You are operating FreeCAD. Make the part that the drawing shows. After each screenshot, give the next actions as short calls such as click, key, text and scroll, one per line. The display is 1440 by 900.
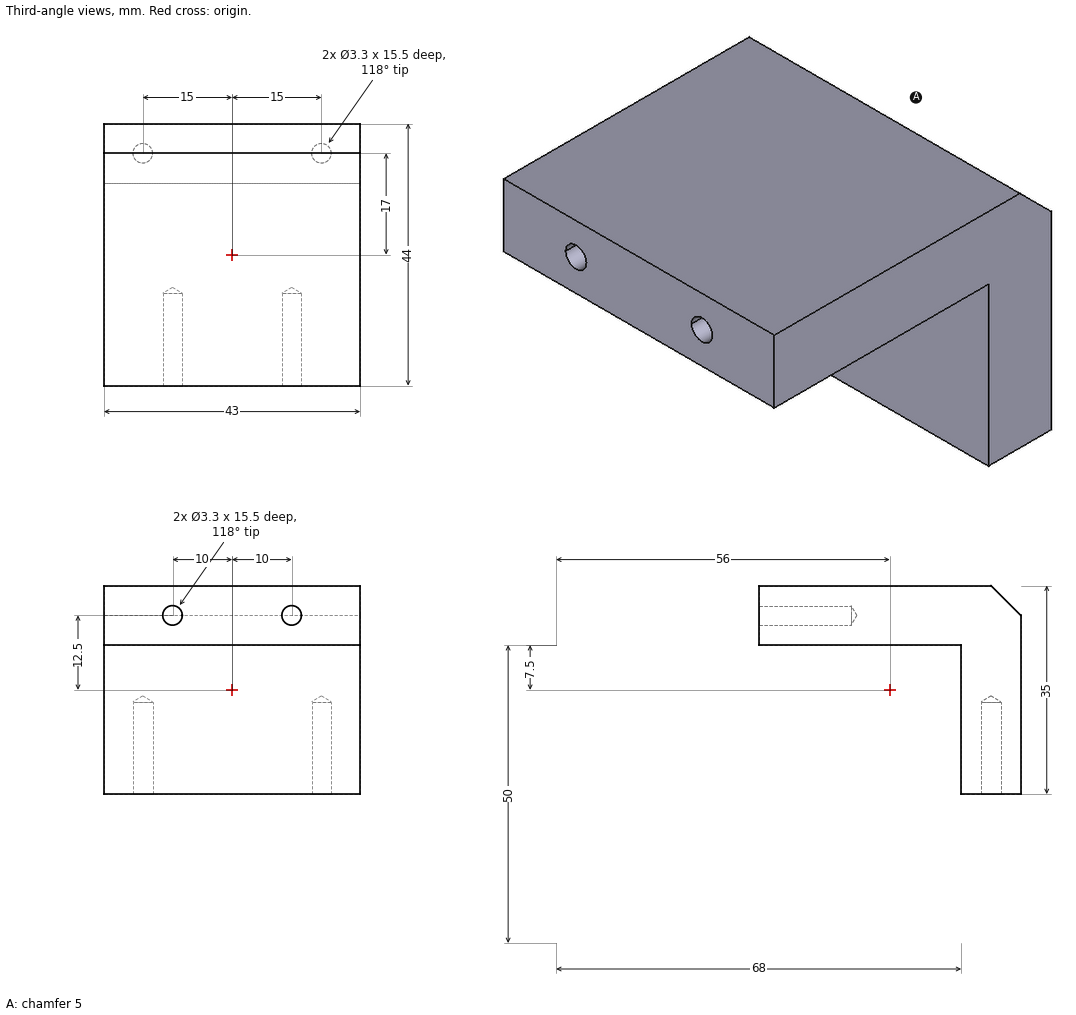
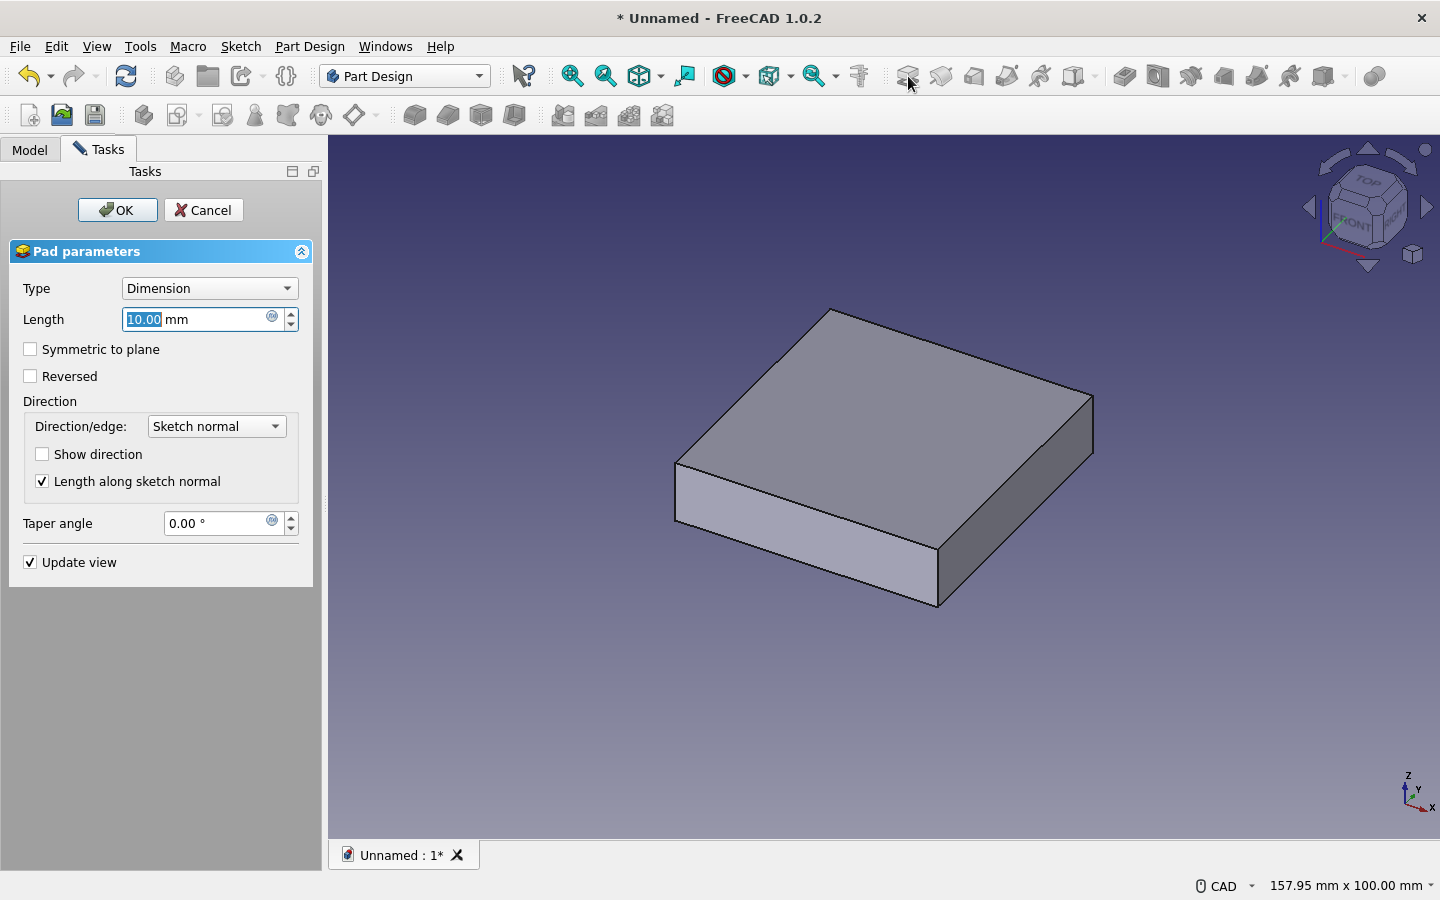
text(35)
key(Tab)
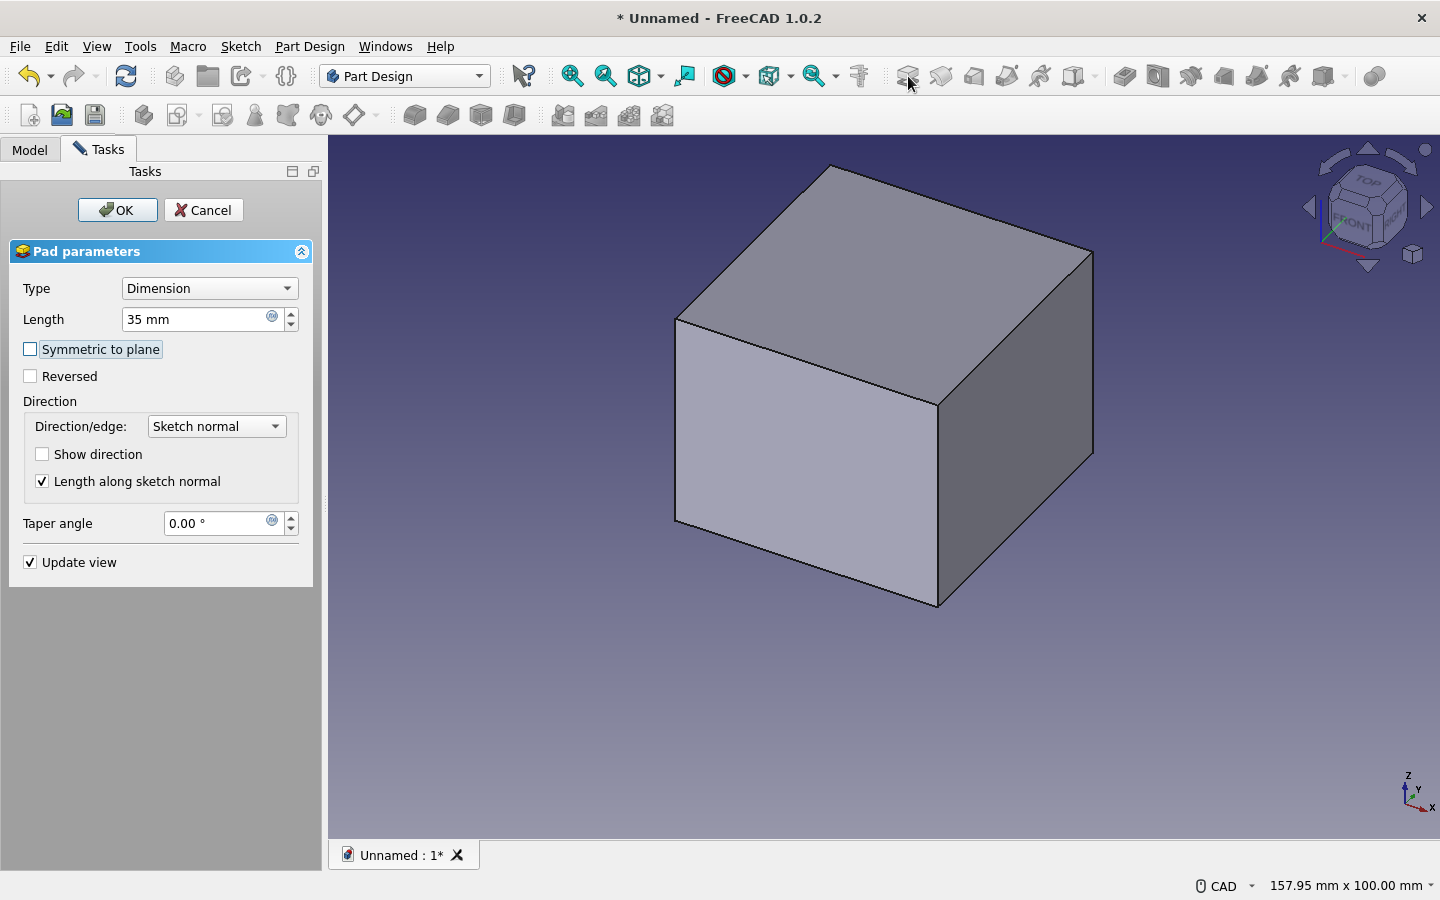
click(31, 349)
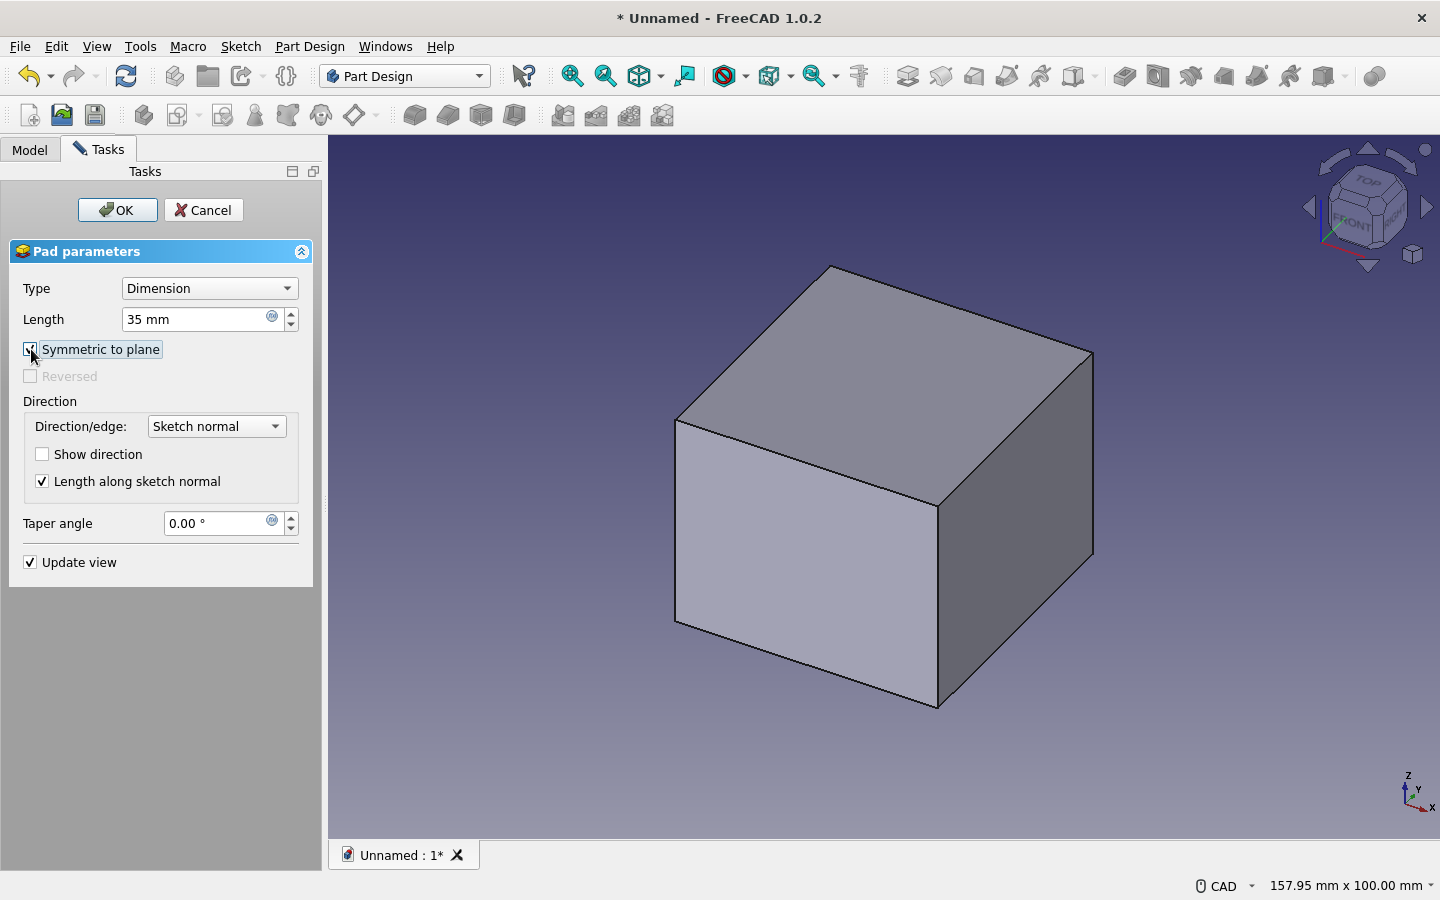
click(118, 210)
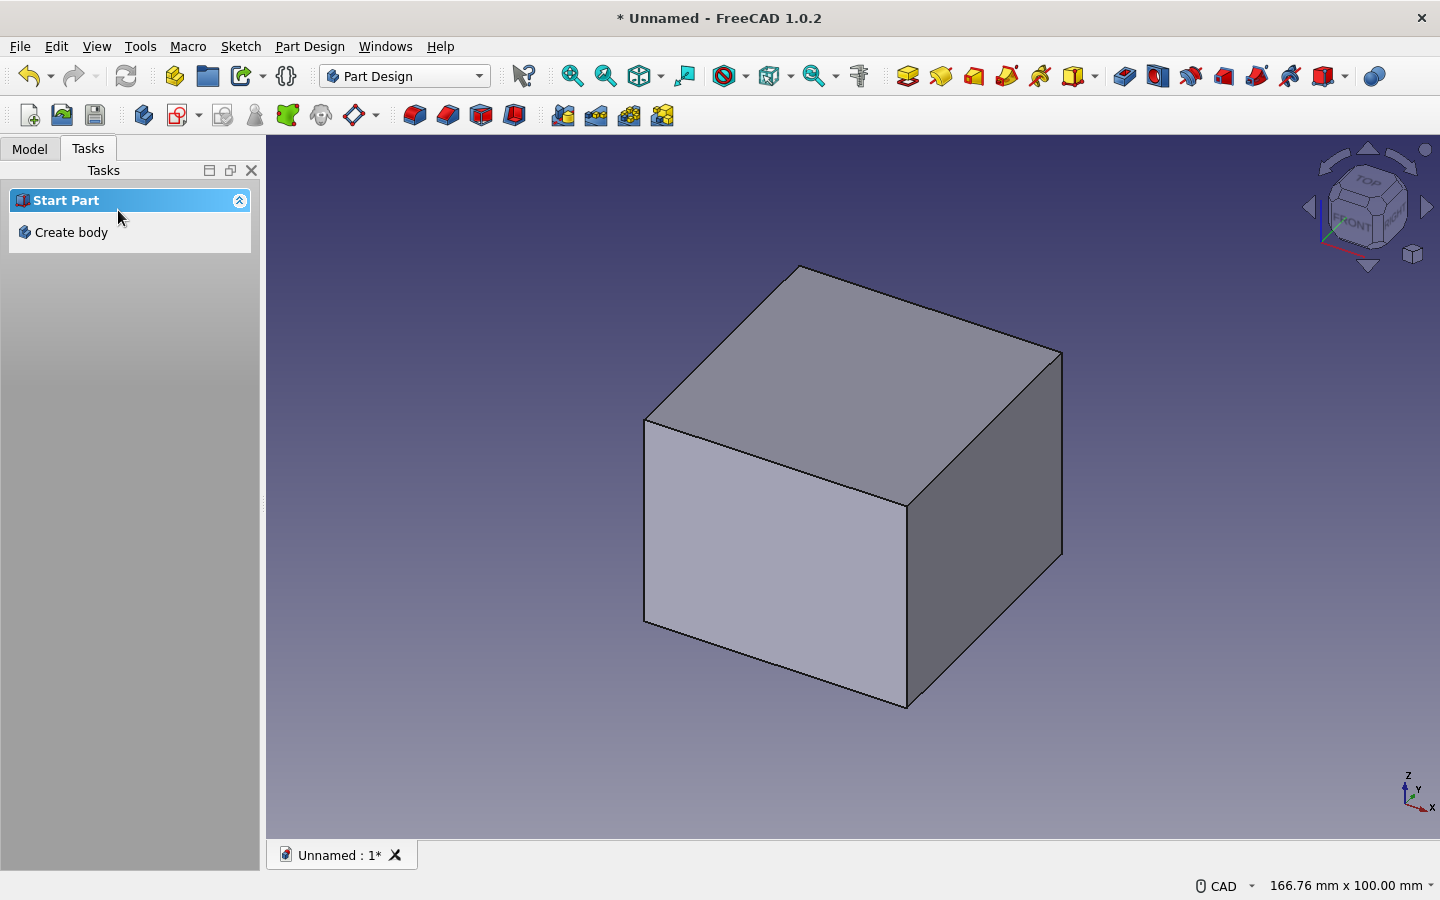
click(984, 529)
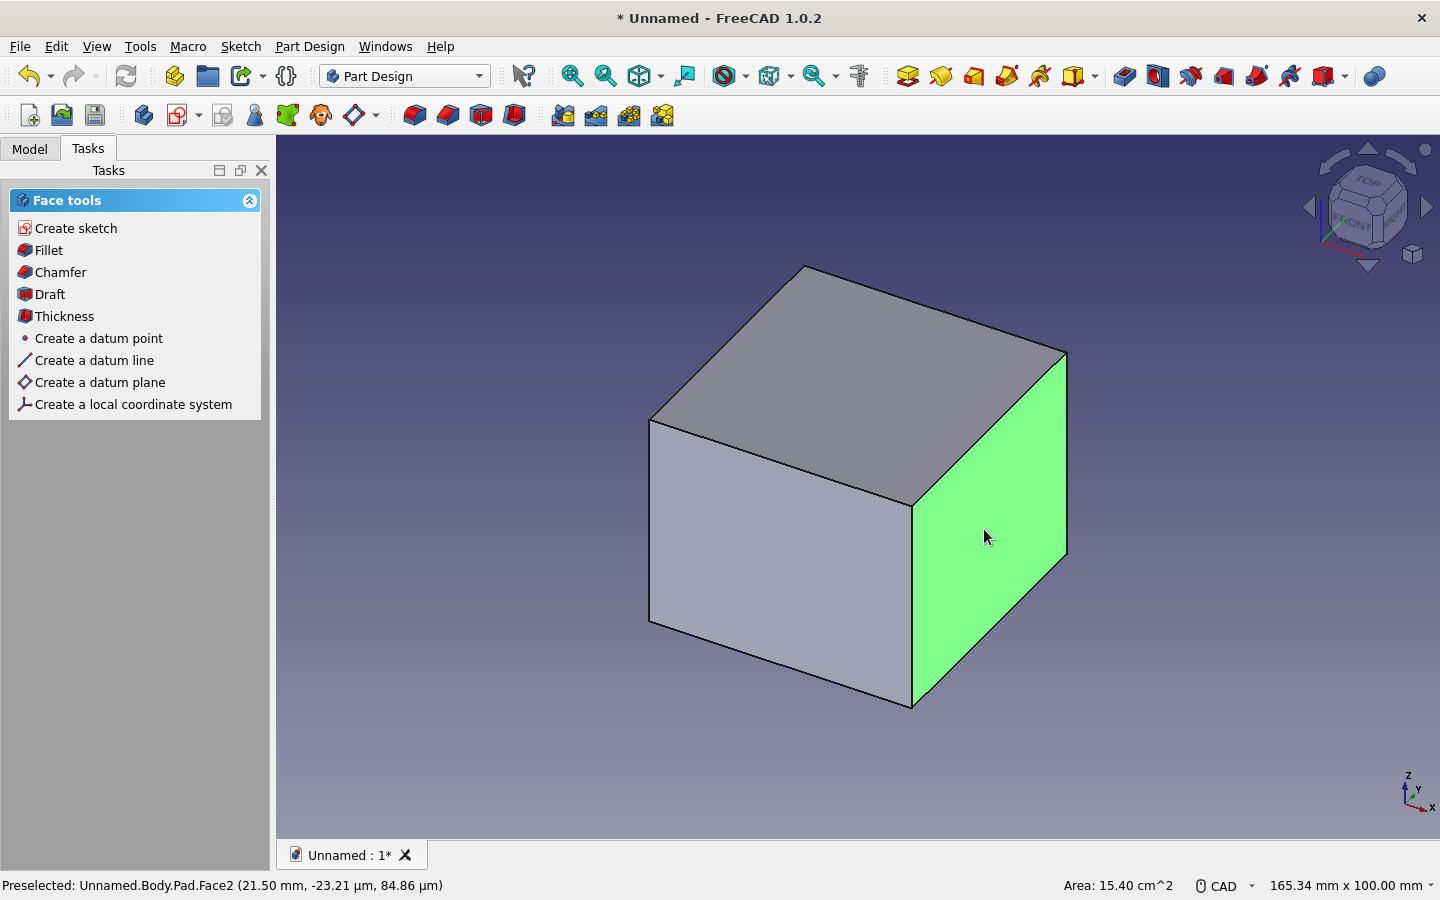
click(176, 116)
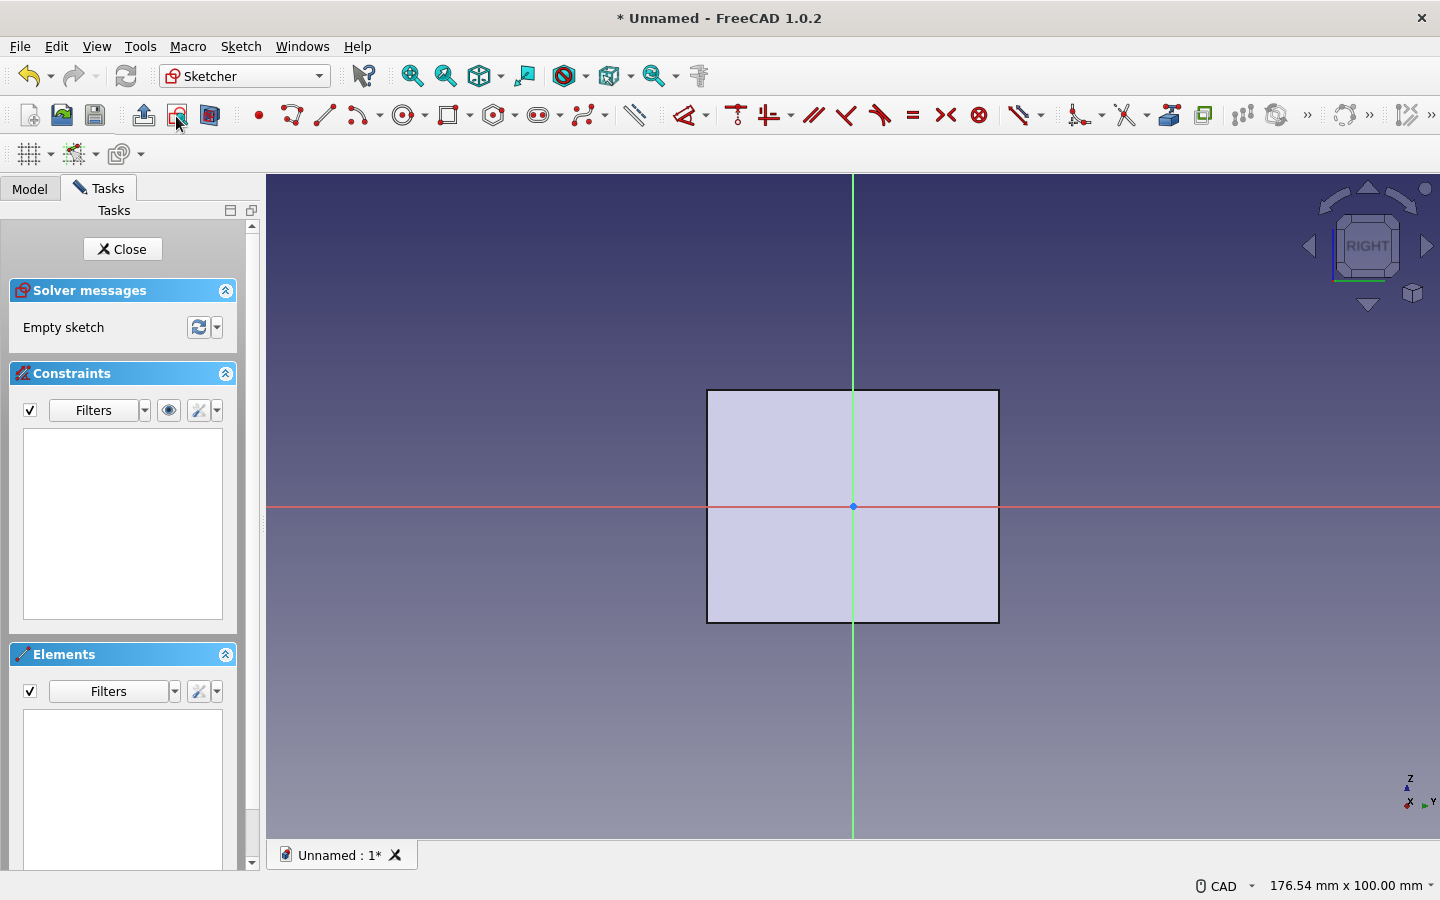
scroll(355, 811, up, 1)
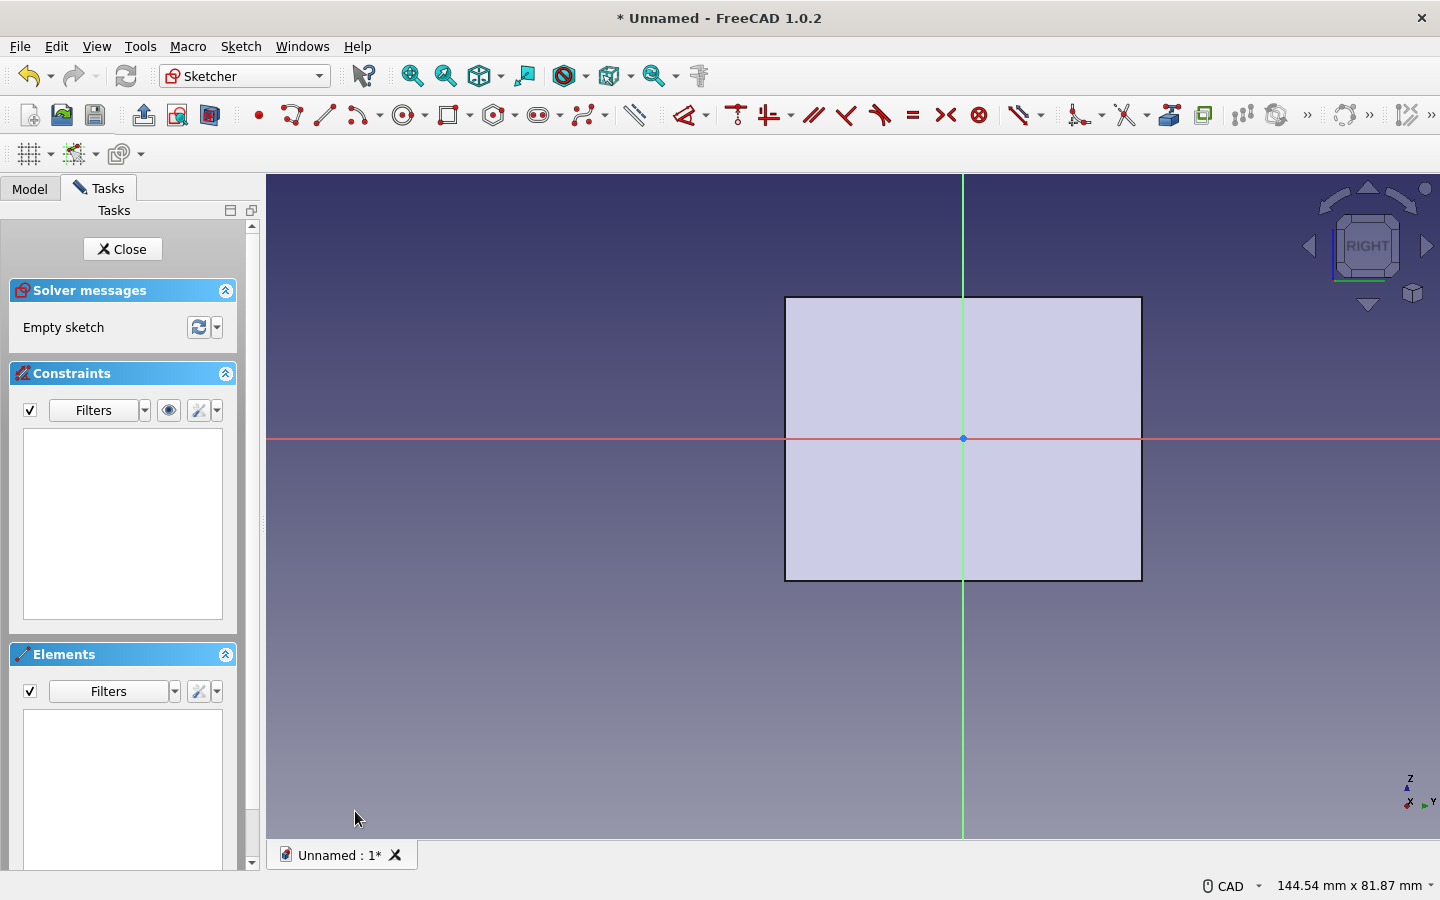
click(448, 116)